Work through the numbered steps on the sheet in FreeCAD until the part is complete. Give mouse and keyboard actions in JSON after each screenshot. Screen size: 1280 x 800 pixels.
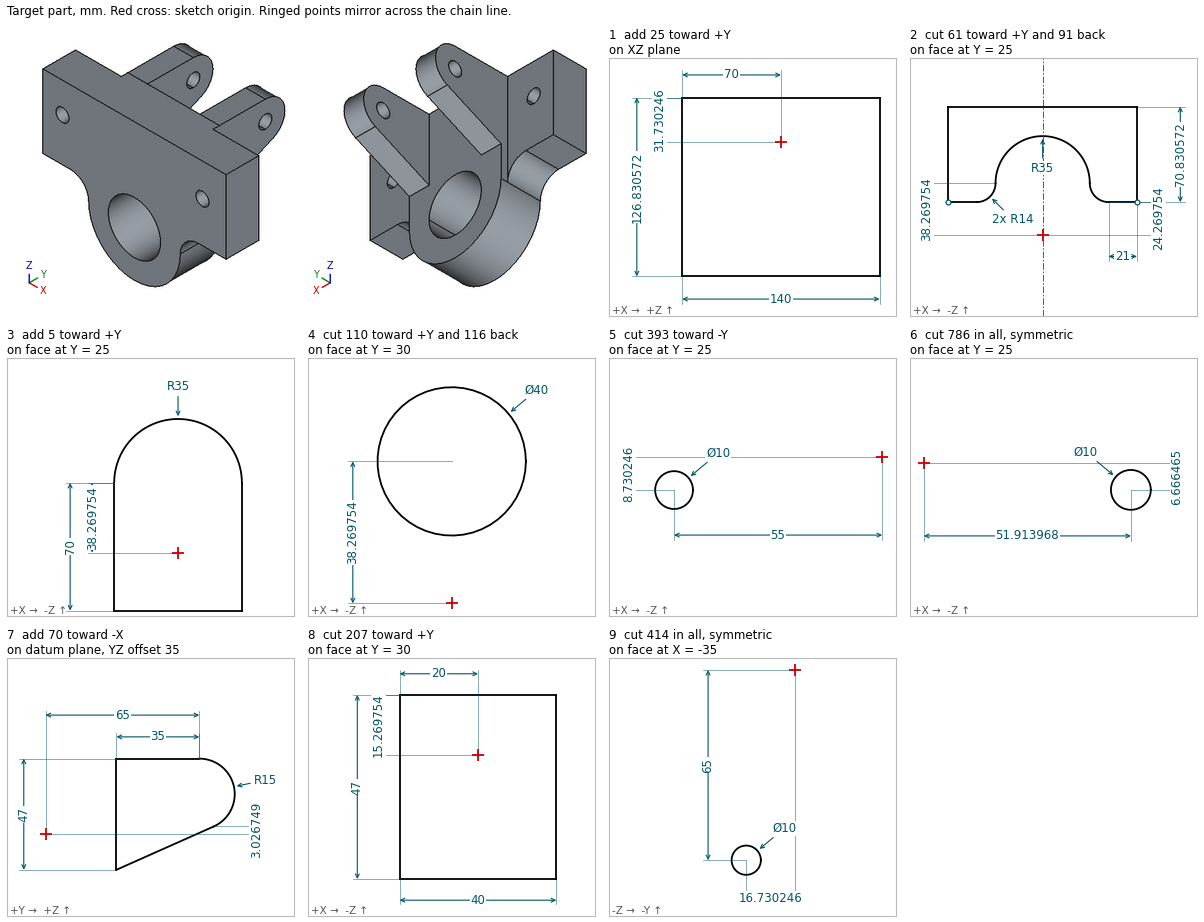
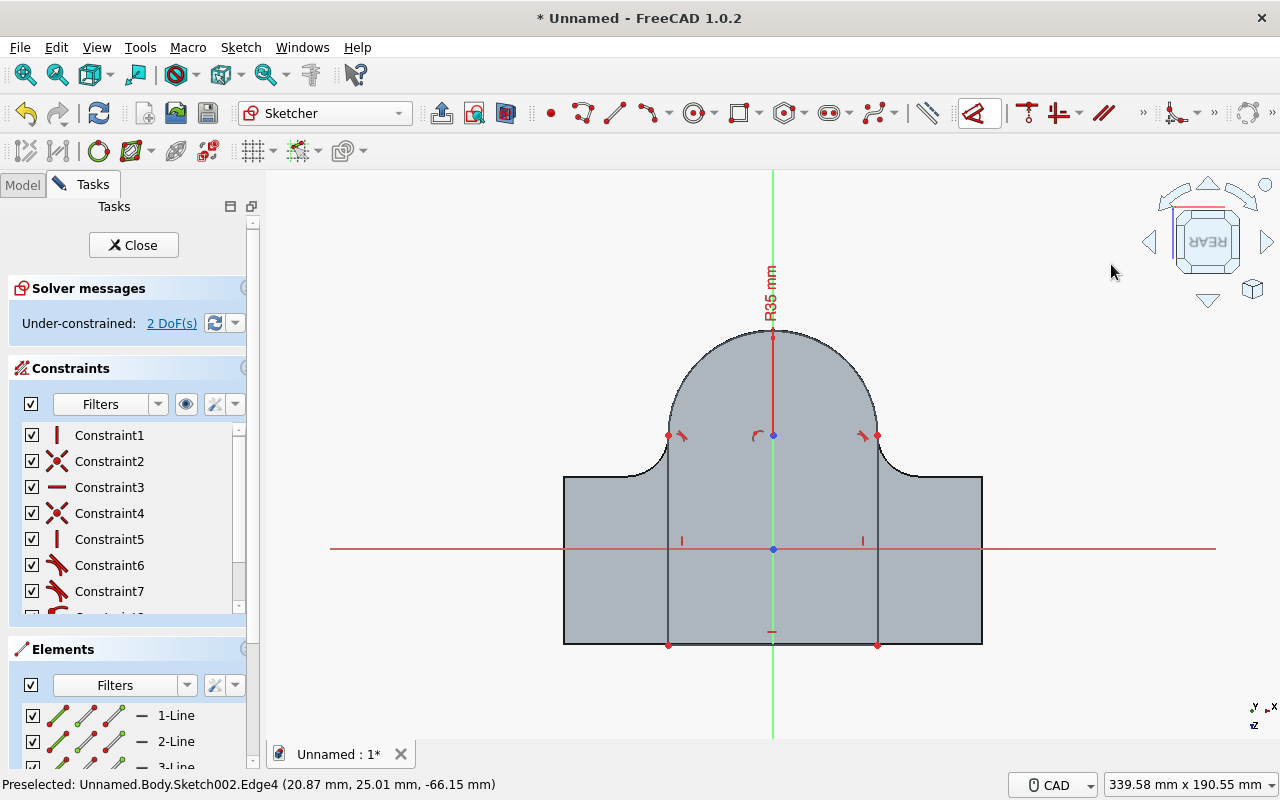
{"action": "left_click", "coordinate": [668, 499]}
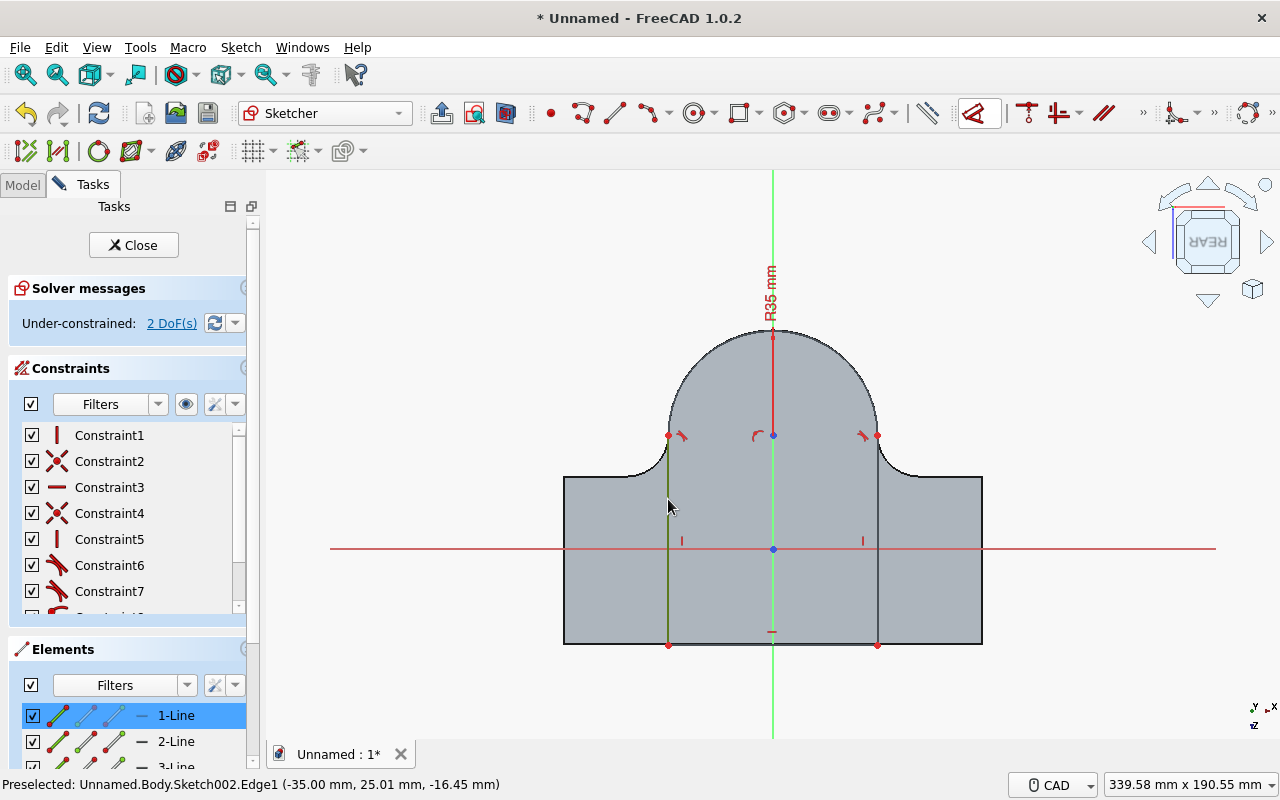
{"action": "left_click", "coordinate": [996, 114]}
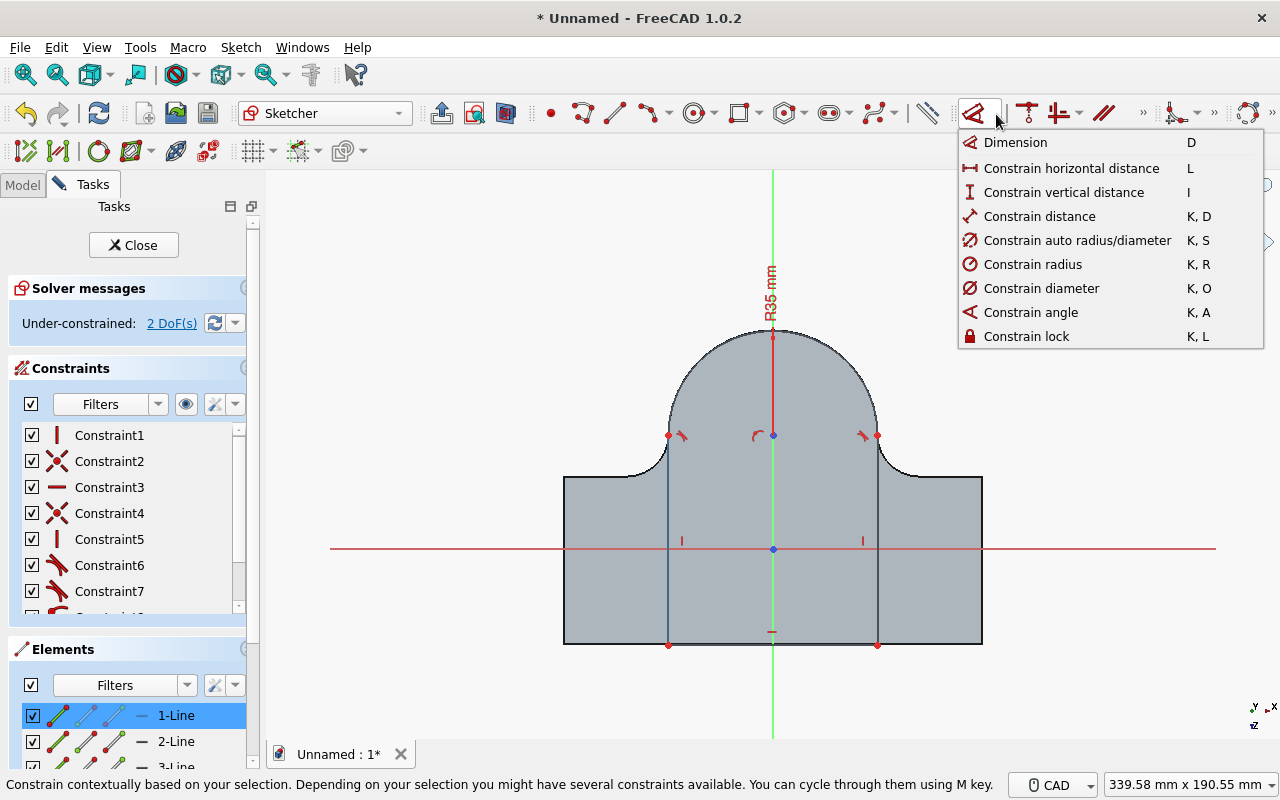
{"action": "left_click", "coordinate": [1111, 192]}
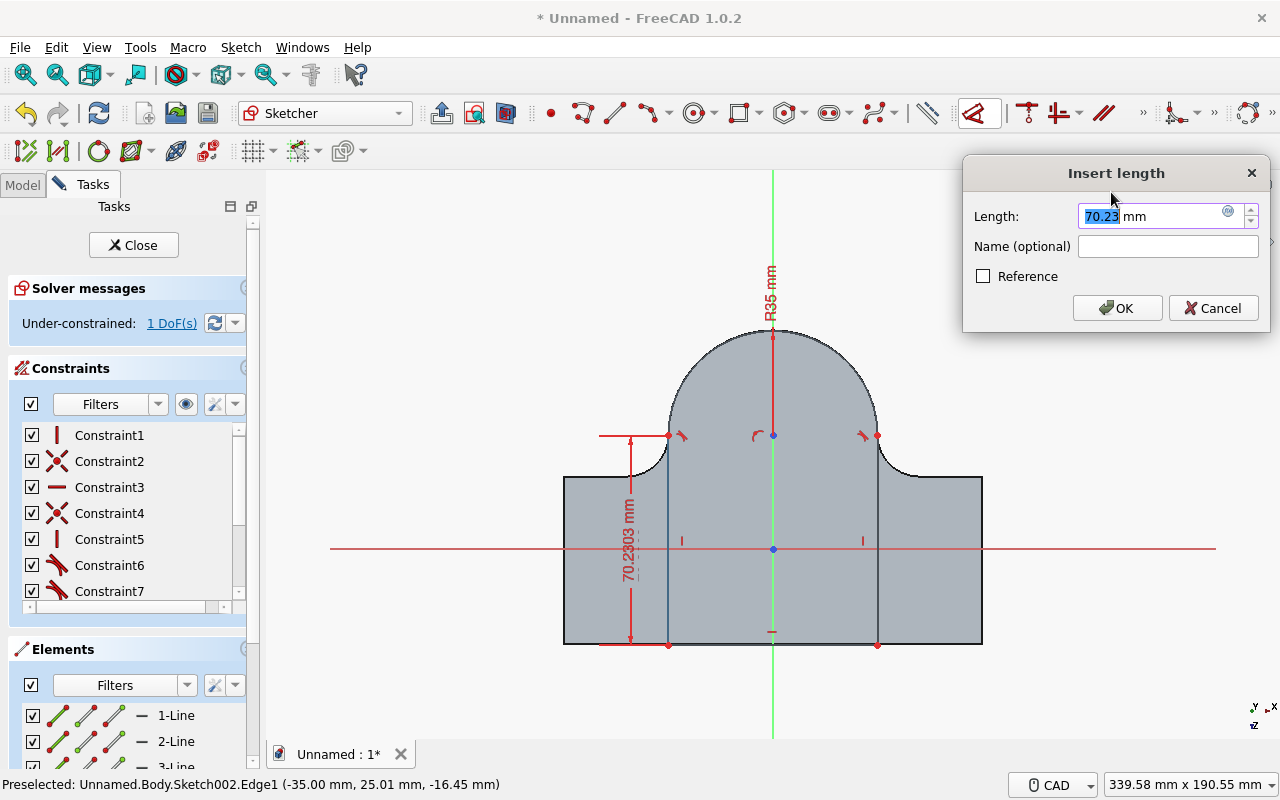
{"action": "type", "text": "70"}
{"action": "key", "text": "Return"}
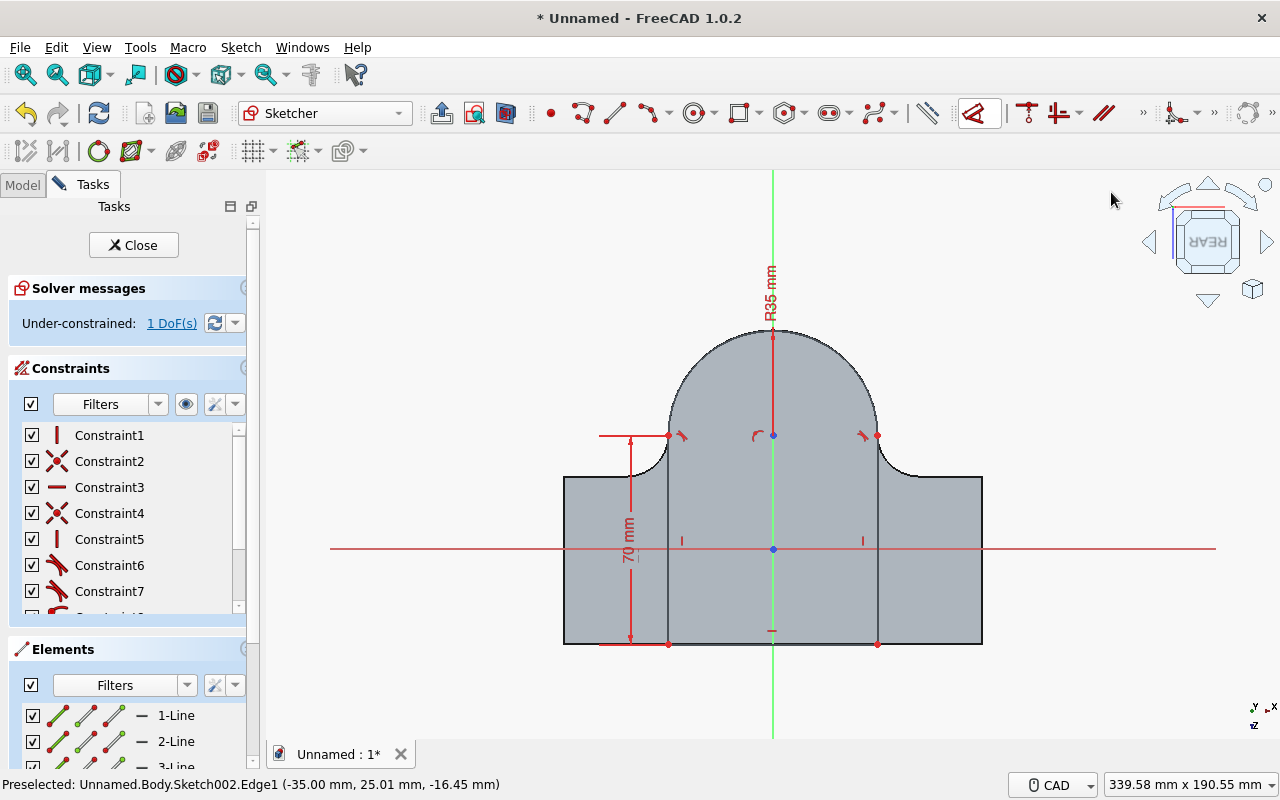
{"action": "left_click", "coordinate": [668, 436]}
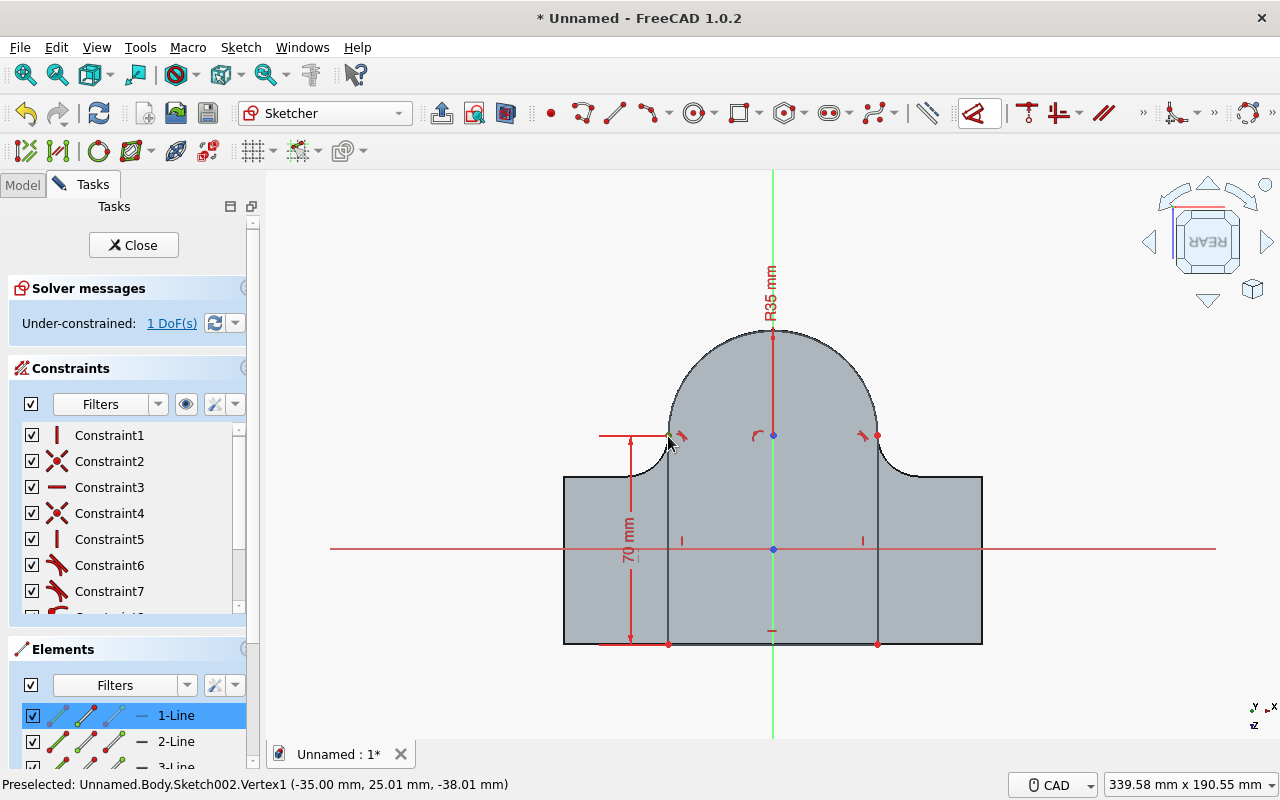
{"action": "key", "text": "i"}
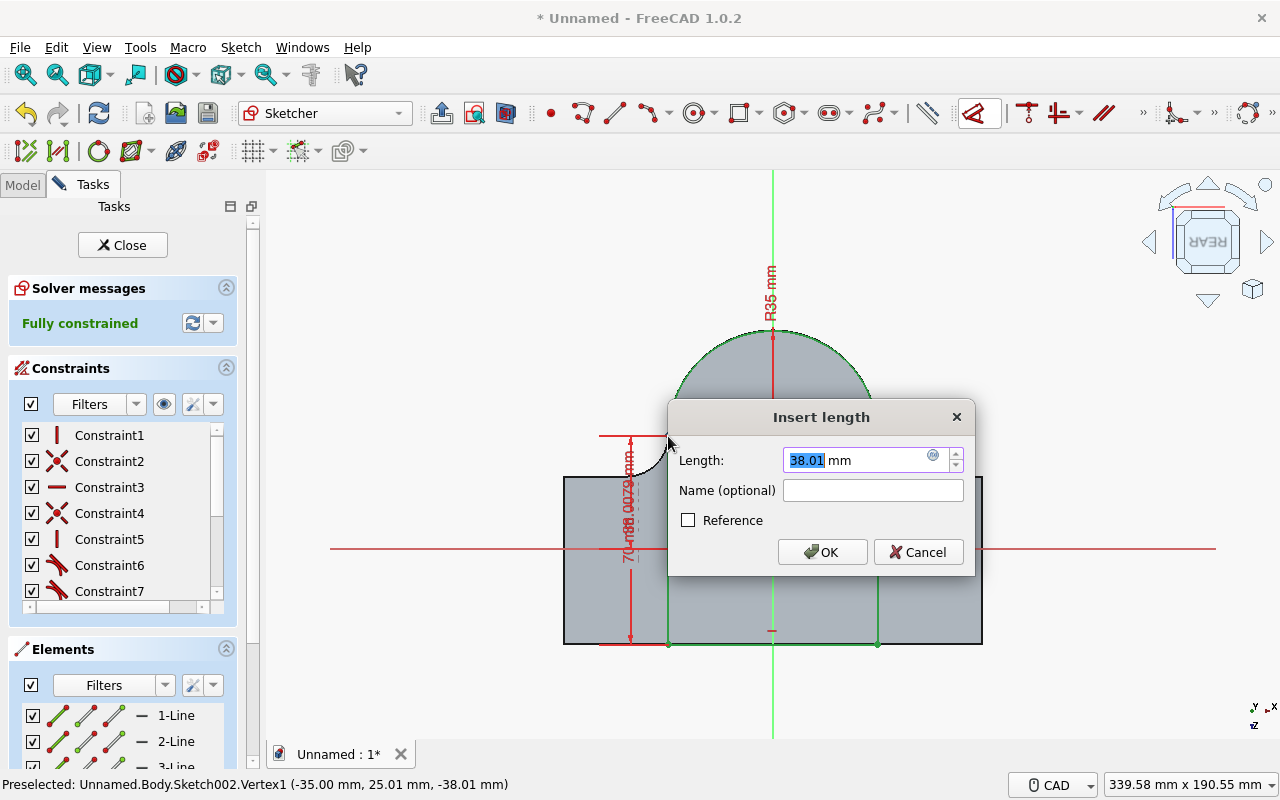
{"action": "type", "text": "38.269754"}
{"action": "key", "text": "Return"}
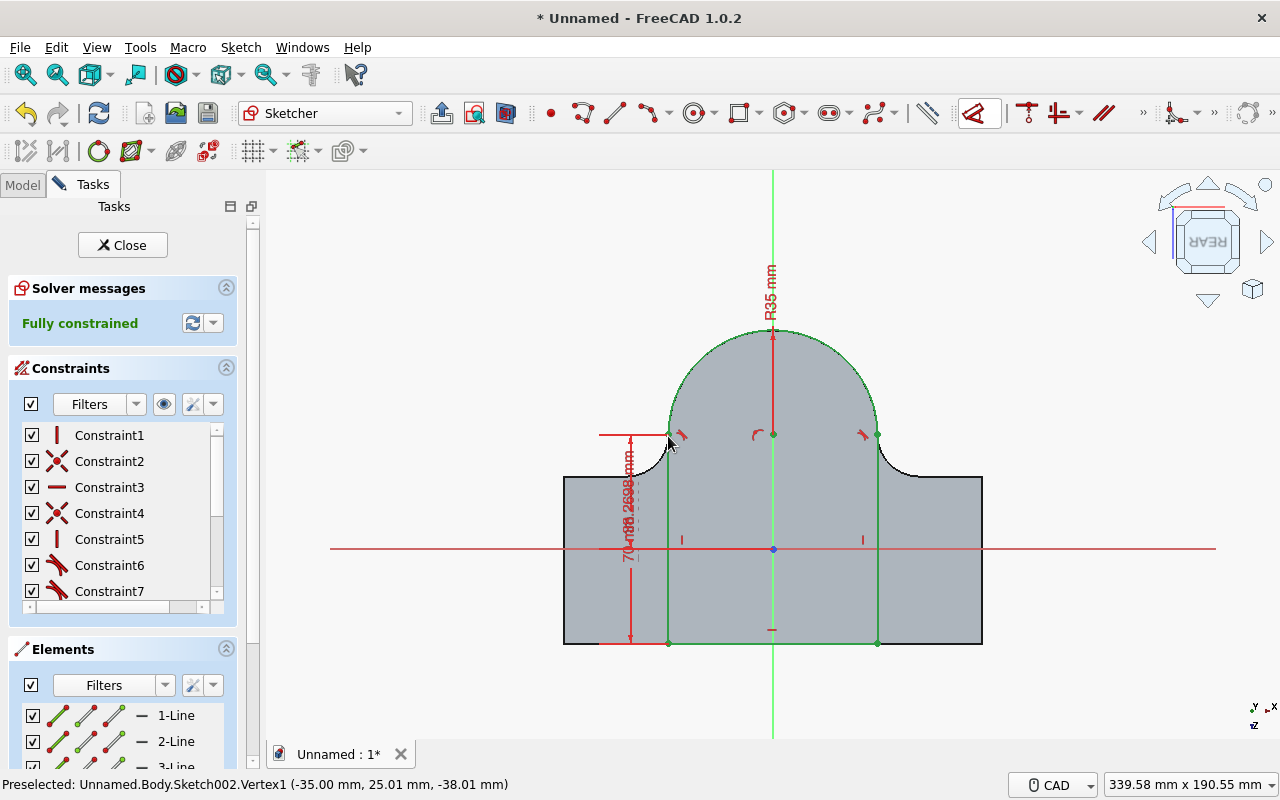
{"action": "left_click", "coordinate": [123, 245]}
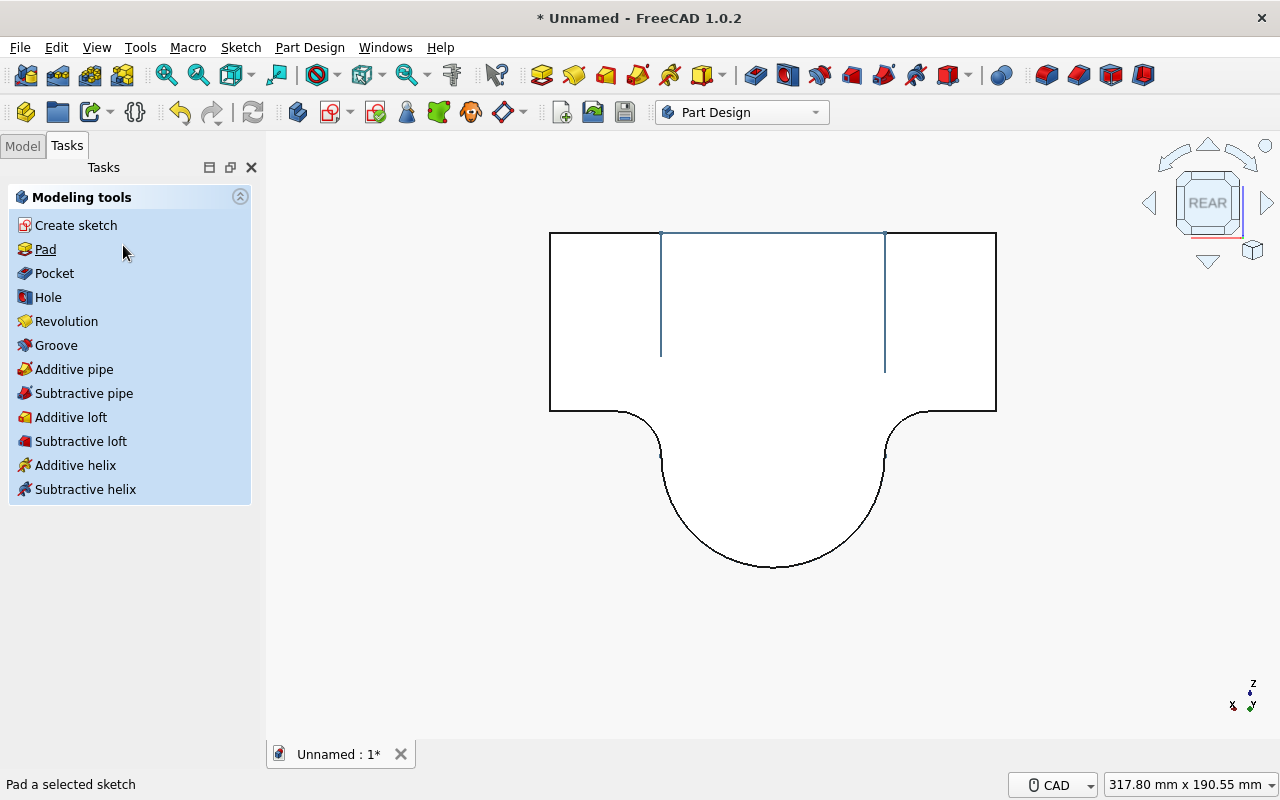
{"action": "left_click", "coordinate": [542, 76]}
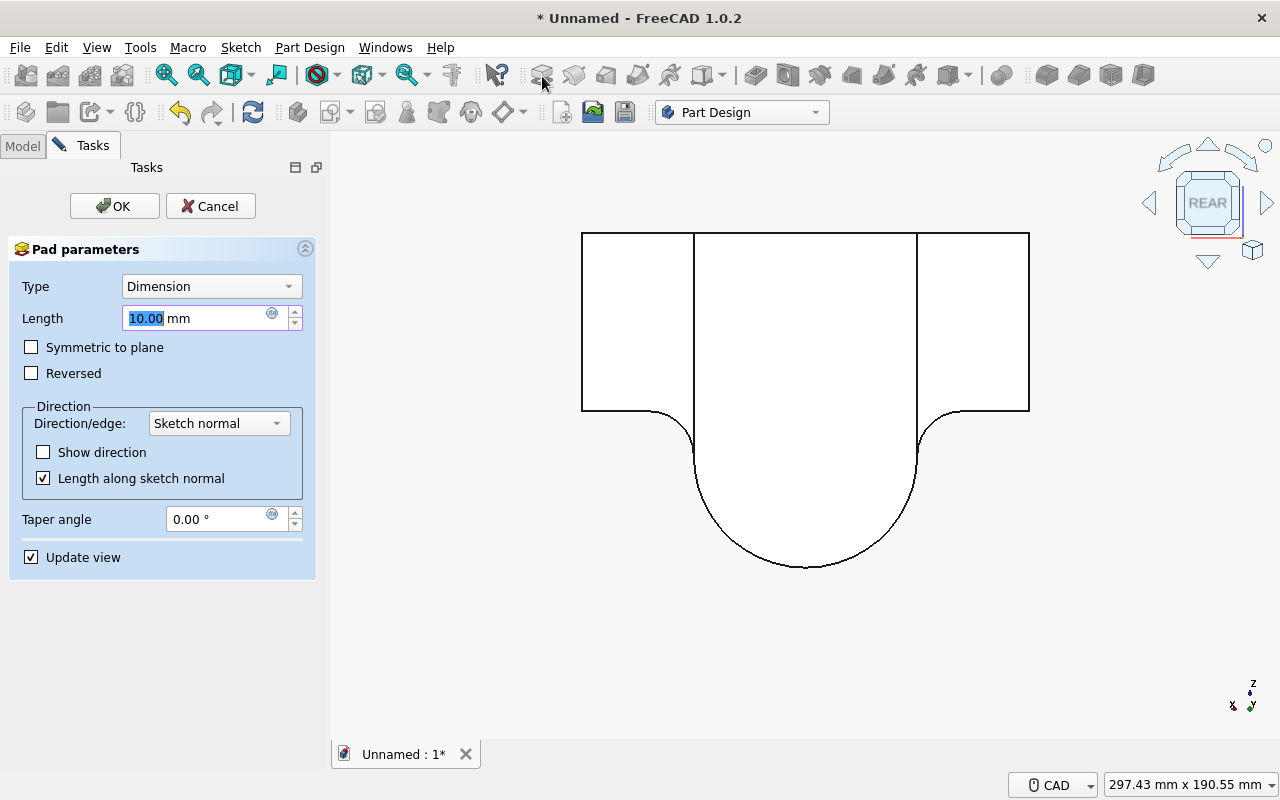
{"action": "type", "text": "5"}
{"action": "key", "text": "Tab"}